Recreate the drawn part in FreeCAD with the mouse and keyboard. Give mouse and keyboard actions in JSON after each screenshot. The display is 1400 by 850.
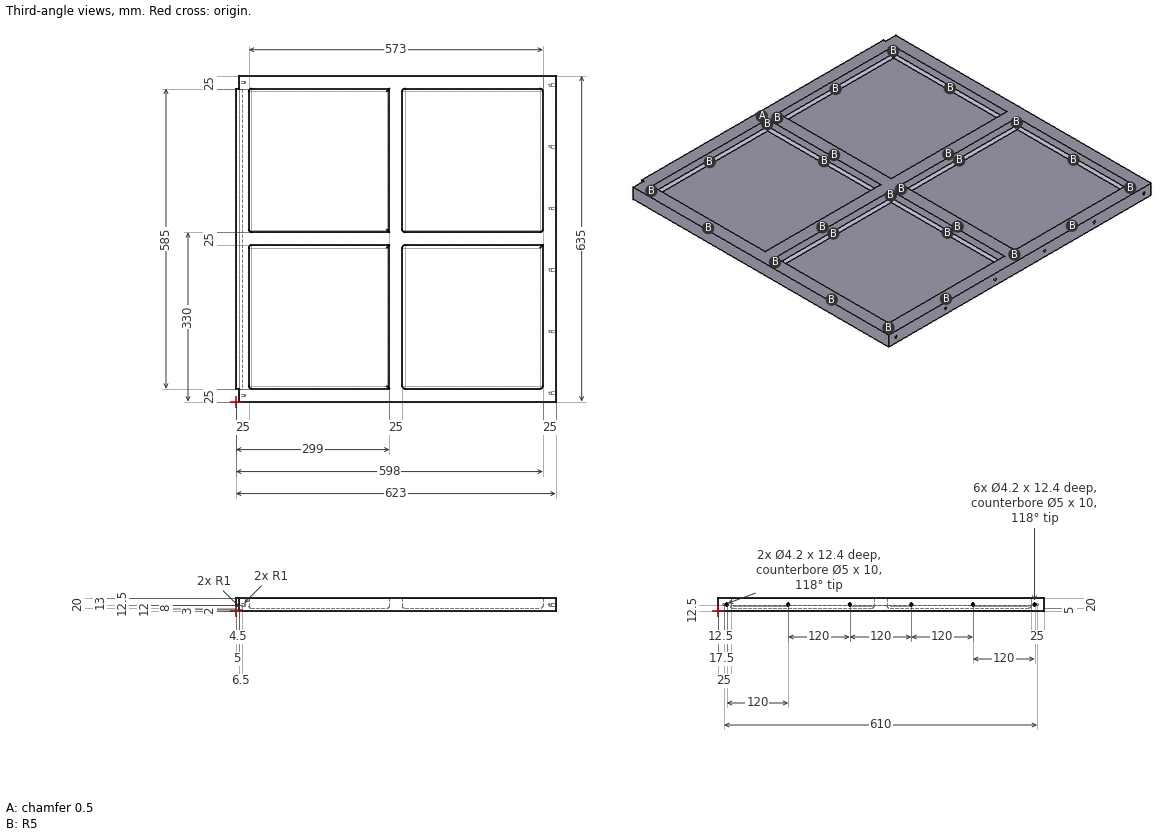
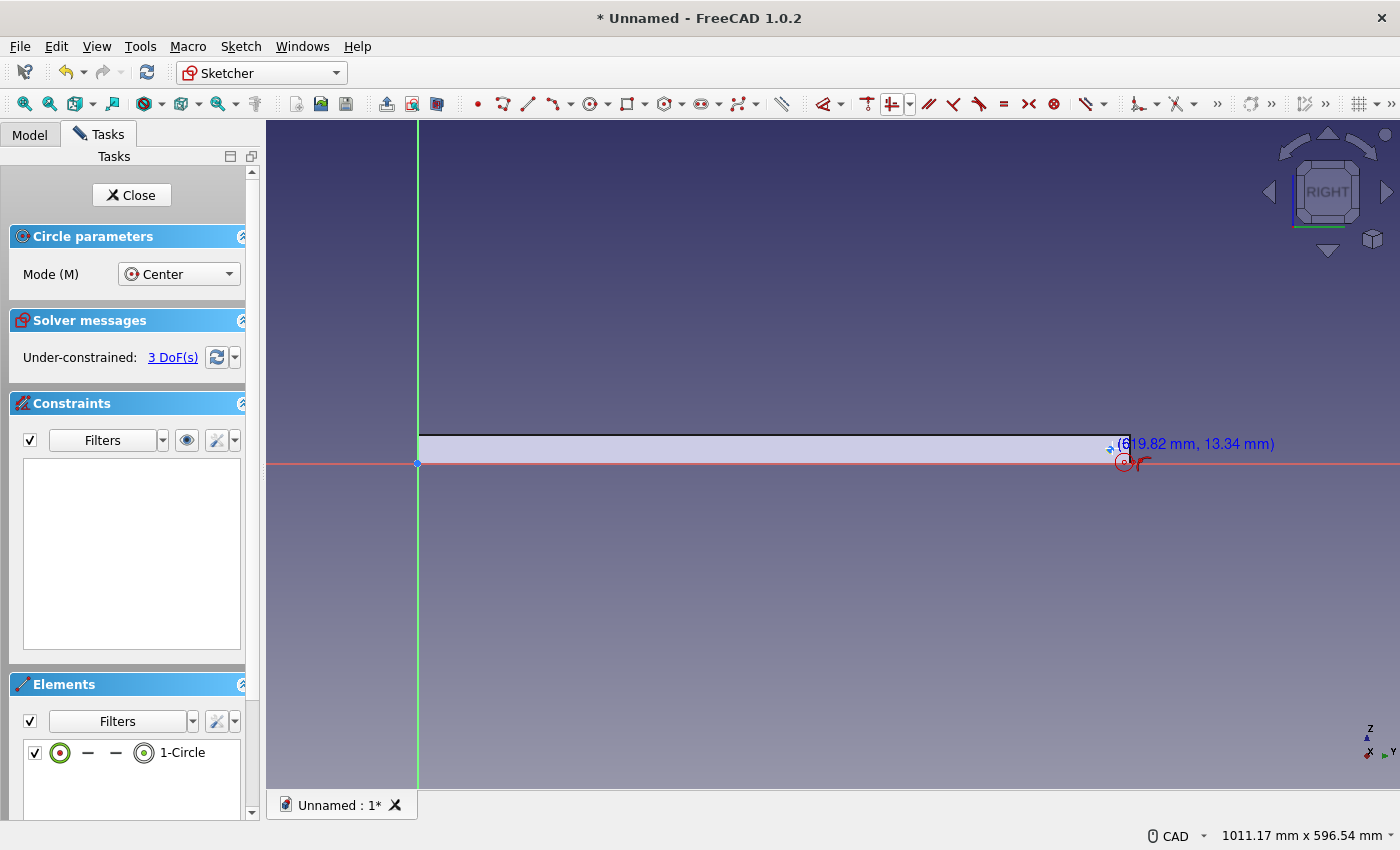
{"action": "scroll", "coordinate": [975, 449], "scroll_direction": "up", "scroll_amount": 12}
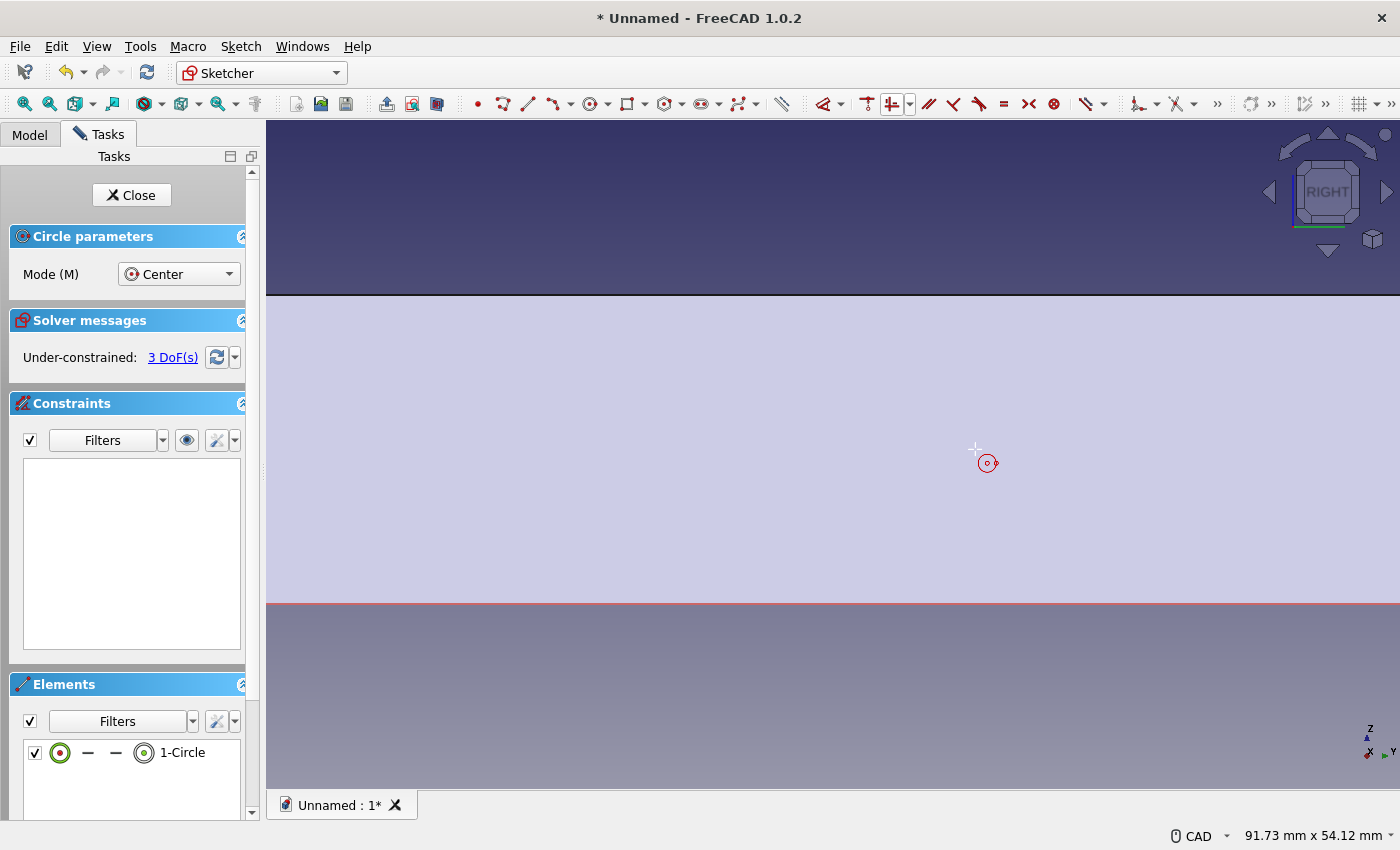
{"action": "scroll", "coordinate": [975, 449], "scroll_direction": "down", "scroll_amount": 12}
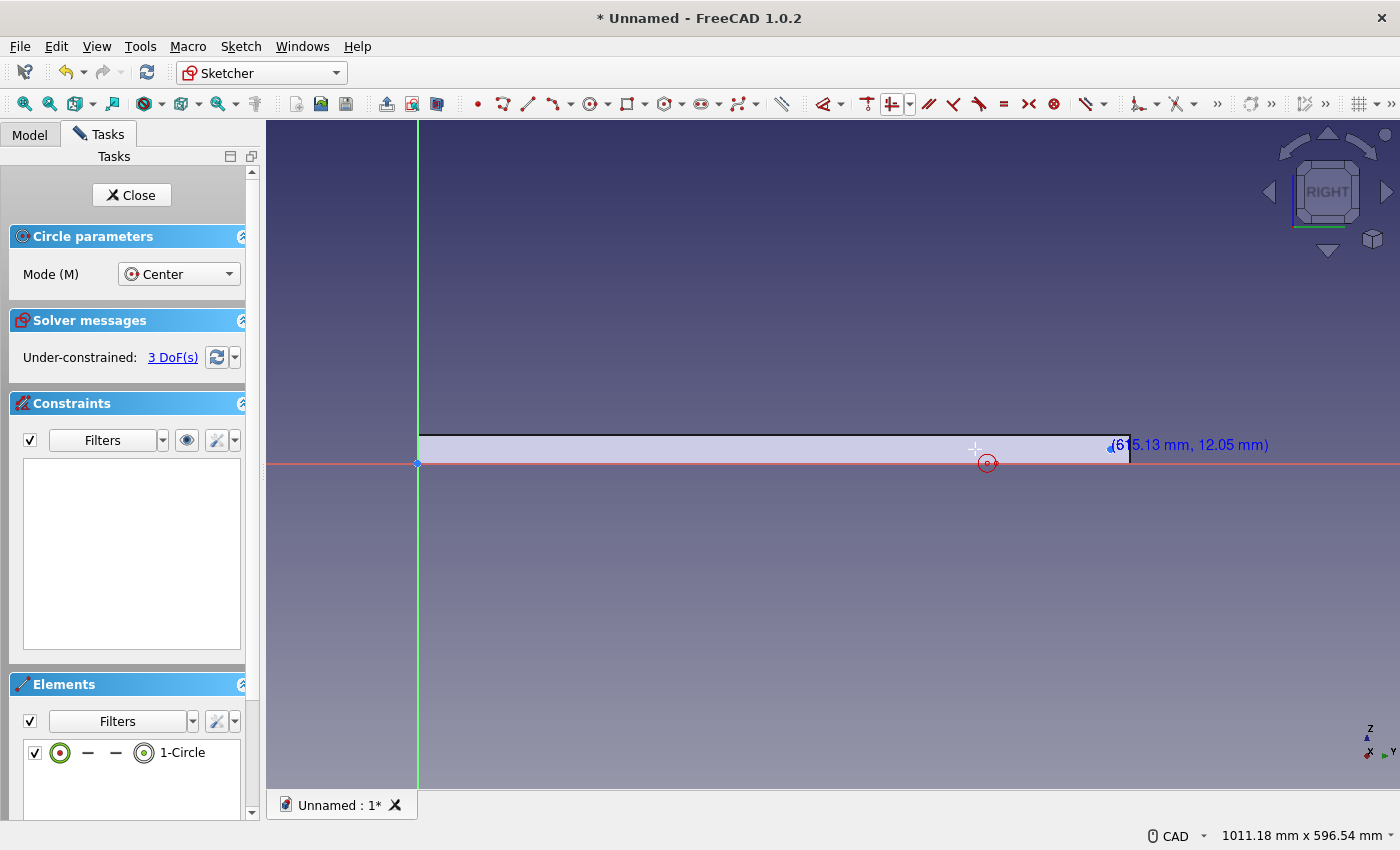
{"action": "left_click", "coordinate": [975, 449]}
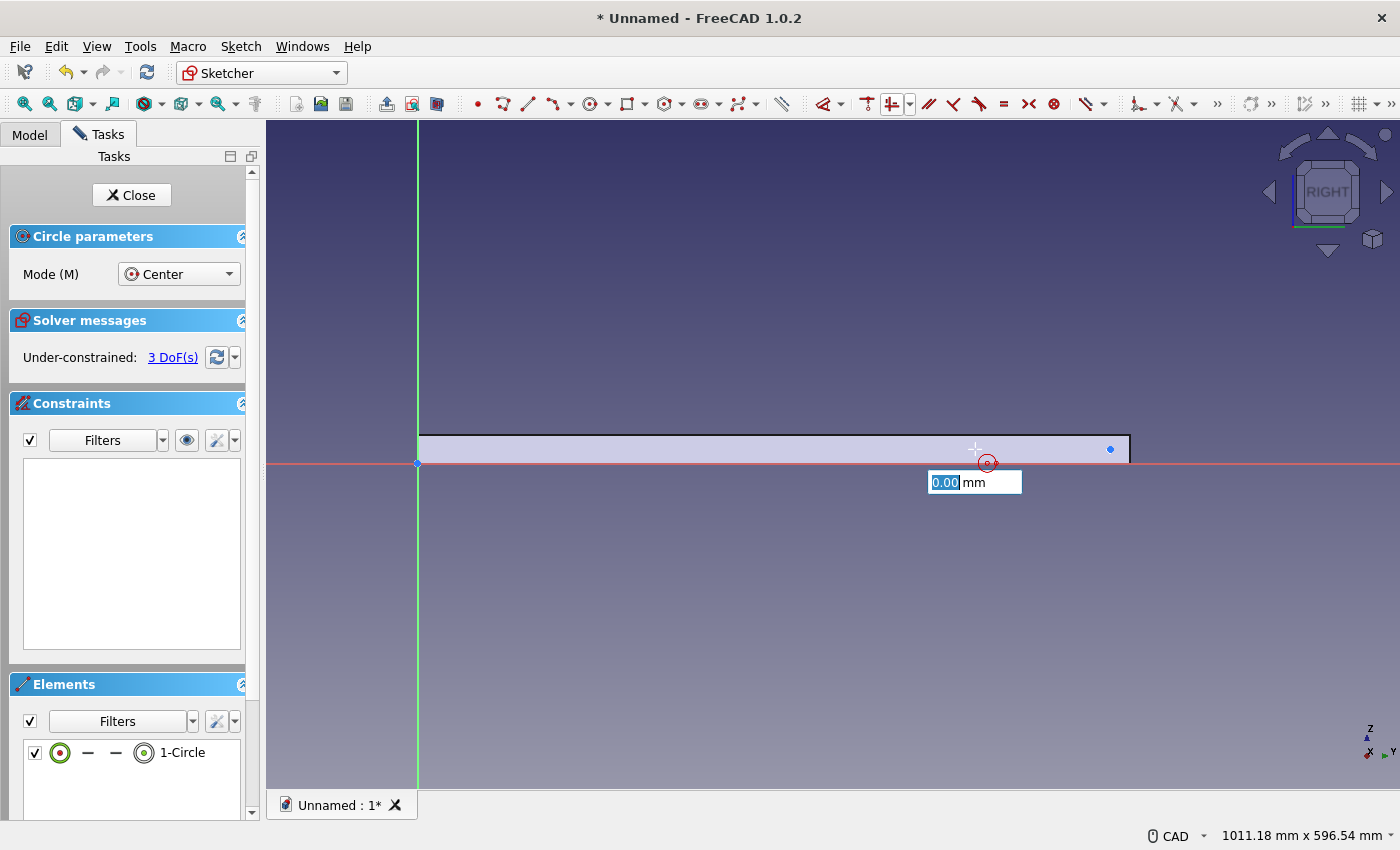
{"action": "scroll", "coordinate": [977, 448], "scroll_direction": "up", "scroll_amount": 10}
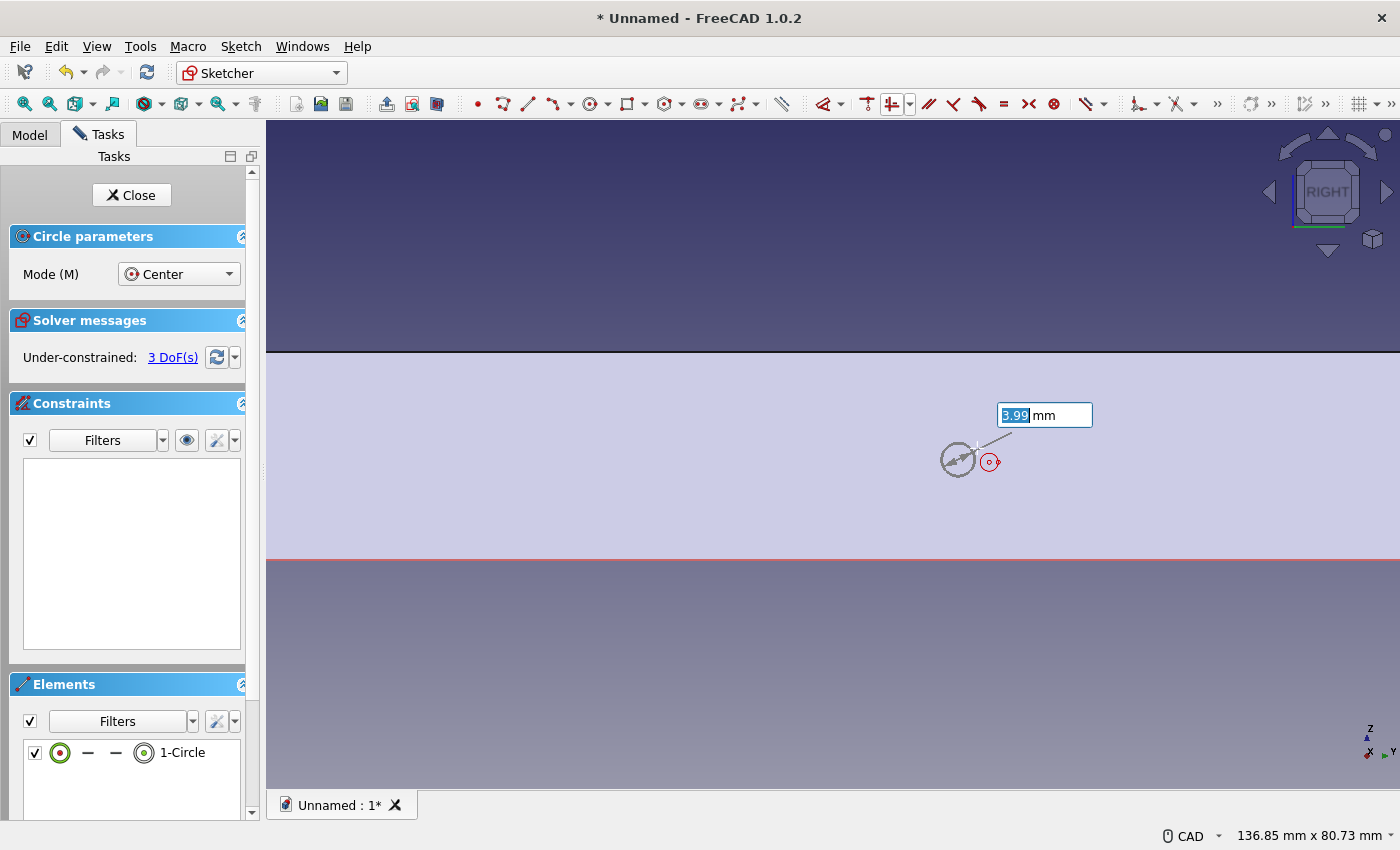
{"action": "left_click", "coordinate": [974, 444]}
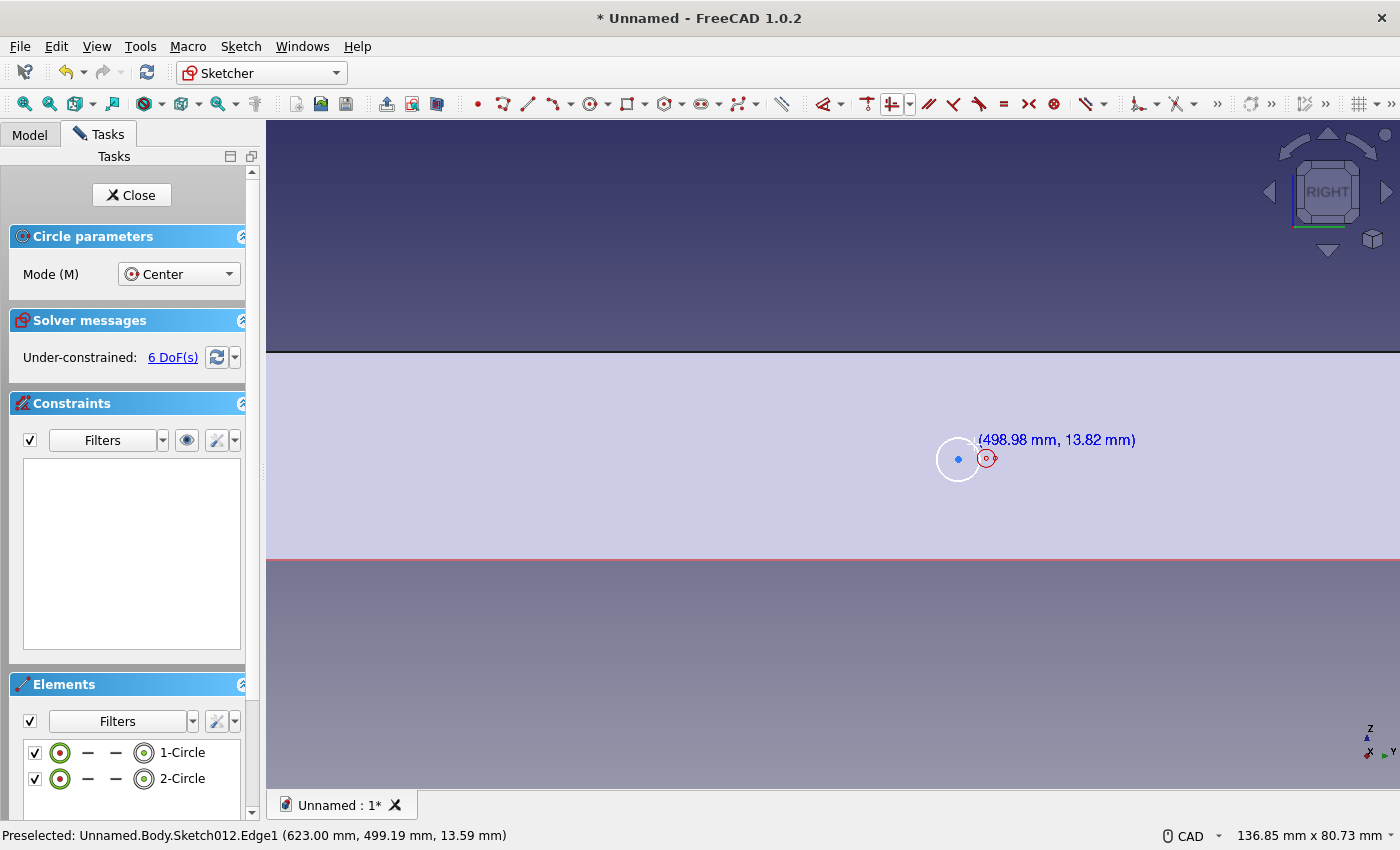
{"action": "scroll", "coordinate": [977, 448], "scroll_direction": "down", "scroll_amount": 10}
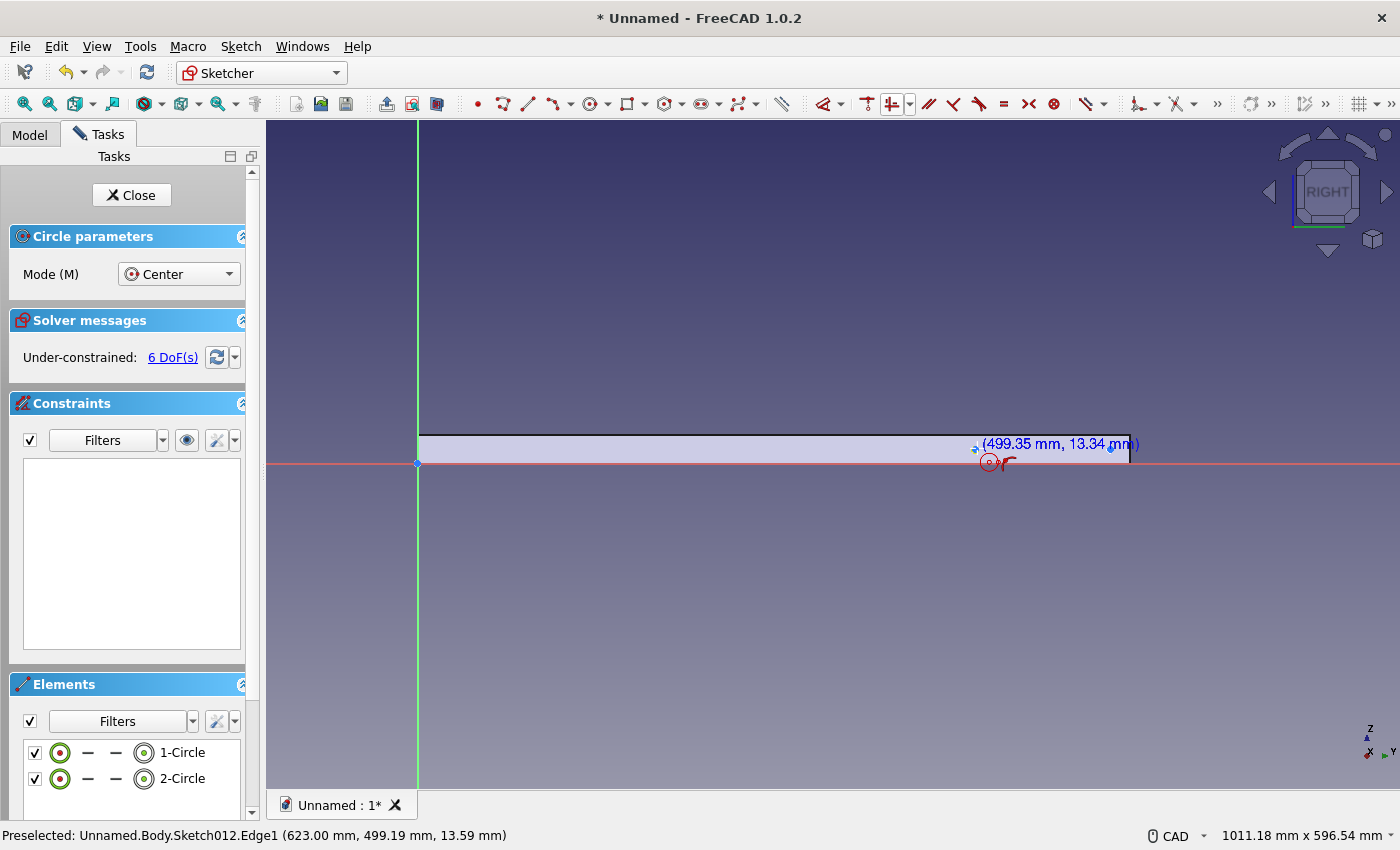
{"action": "scroll", "coordinate": [841, 449], "scroll_direction": "up", "scroll_amount": 12}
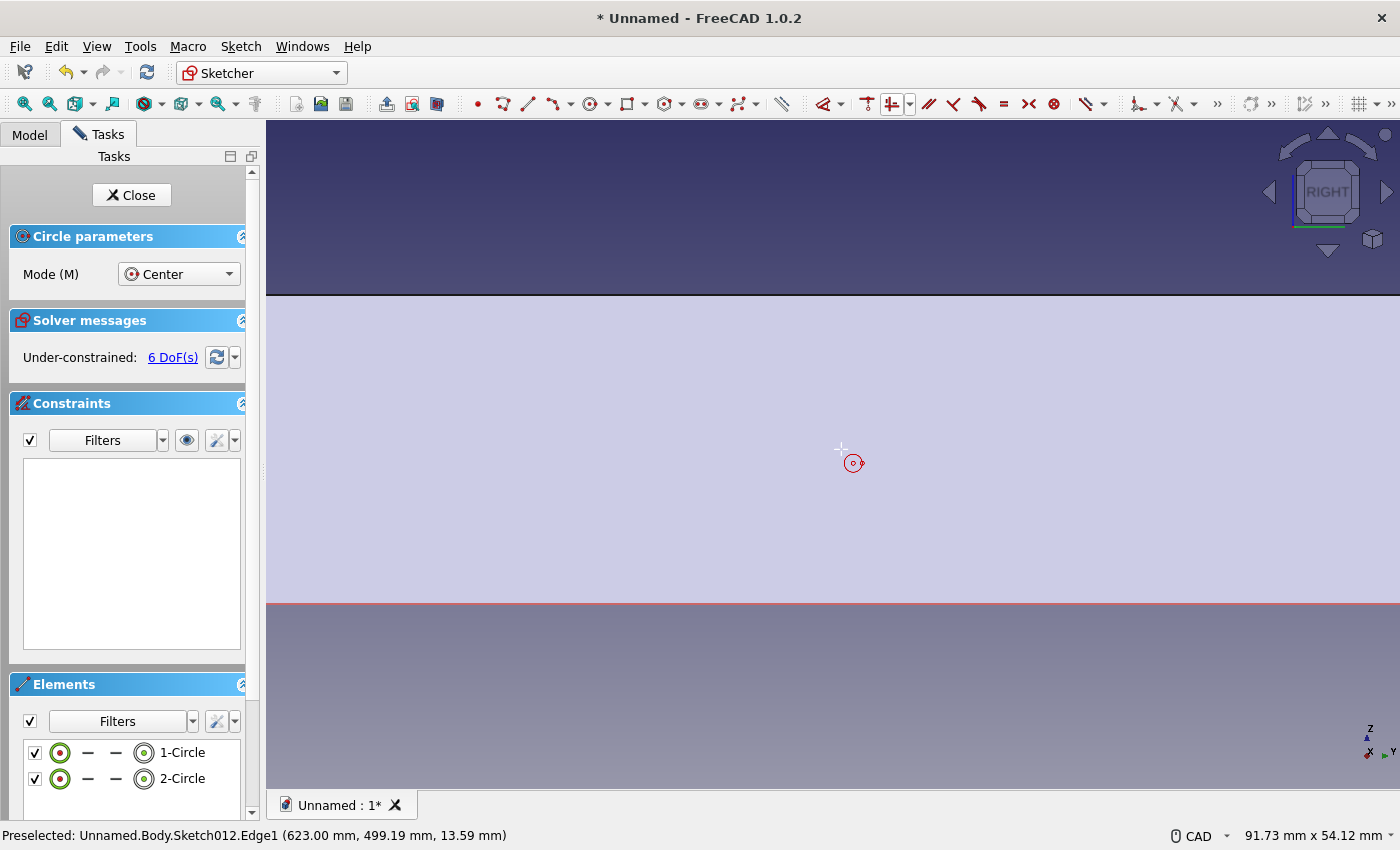
{"action": "scroll", "coordinate": [841, 449], "scroll_direction": "down", "scroll_amount": 12}